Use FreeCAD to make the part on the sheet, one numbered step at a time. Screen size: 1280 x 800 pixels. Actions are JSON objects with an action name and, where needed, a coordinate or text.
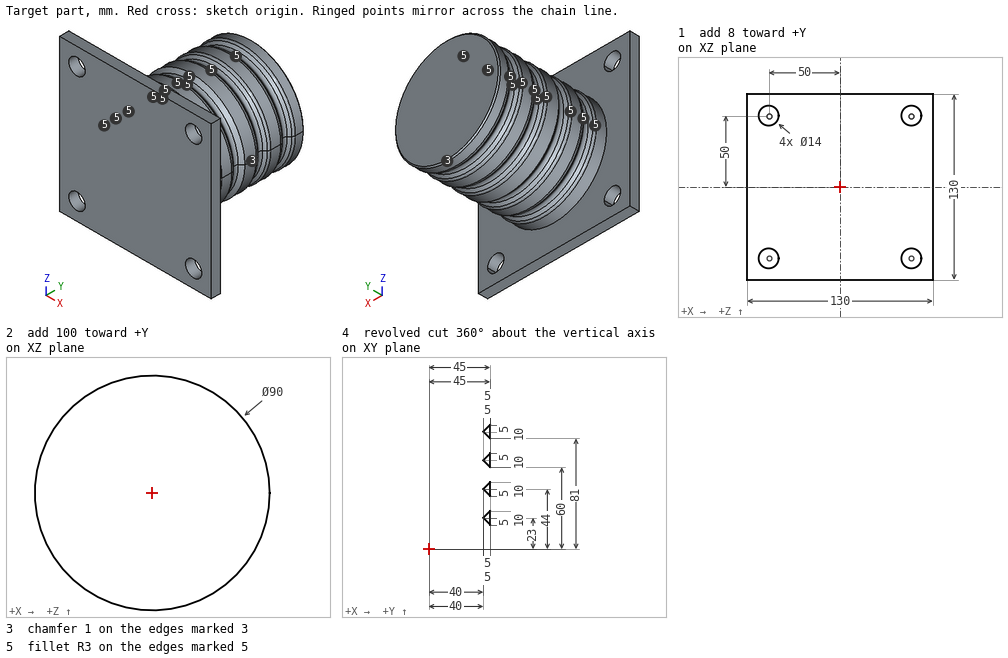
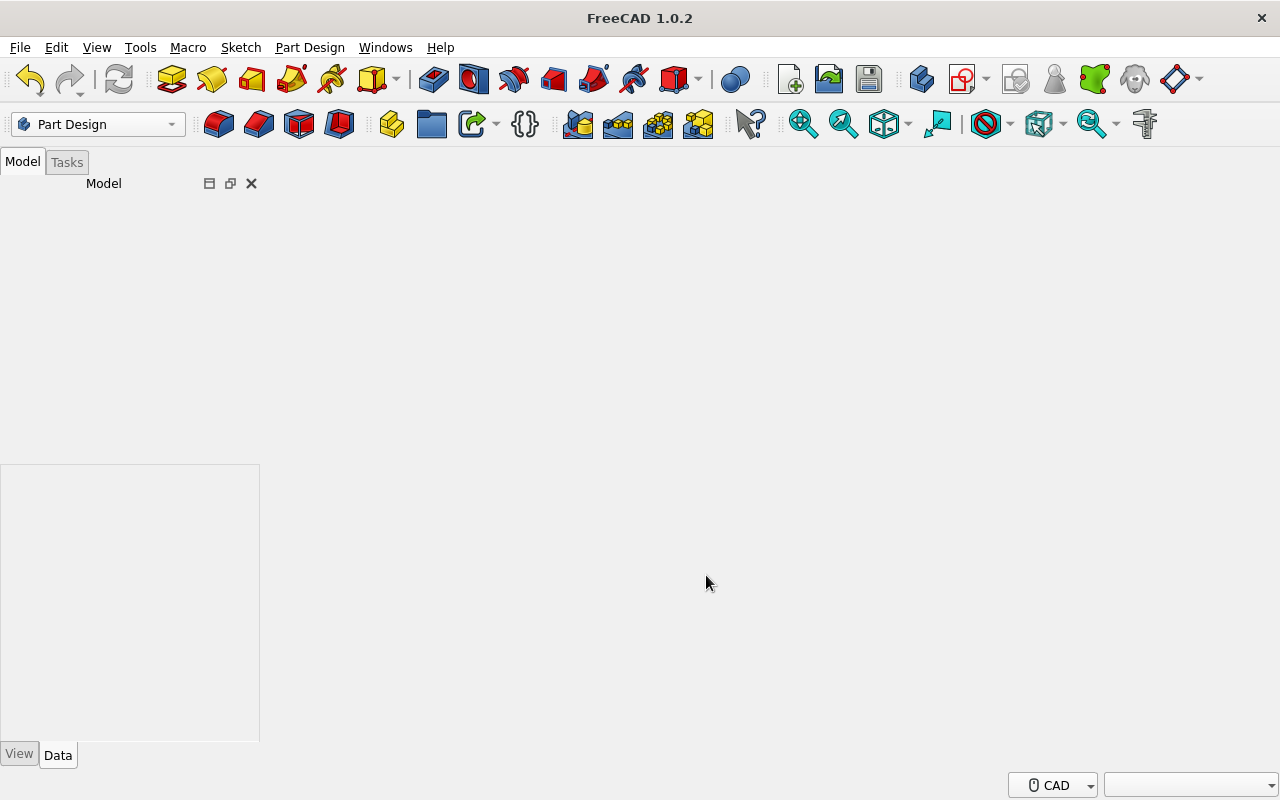
{"action": "left_click", "coordinate": [790, 80]}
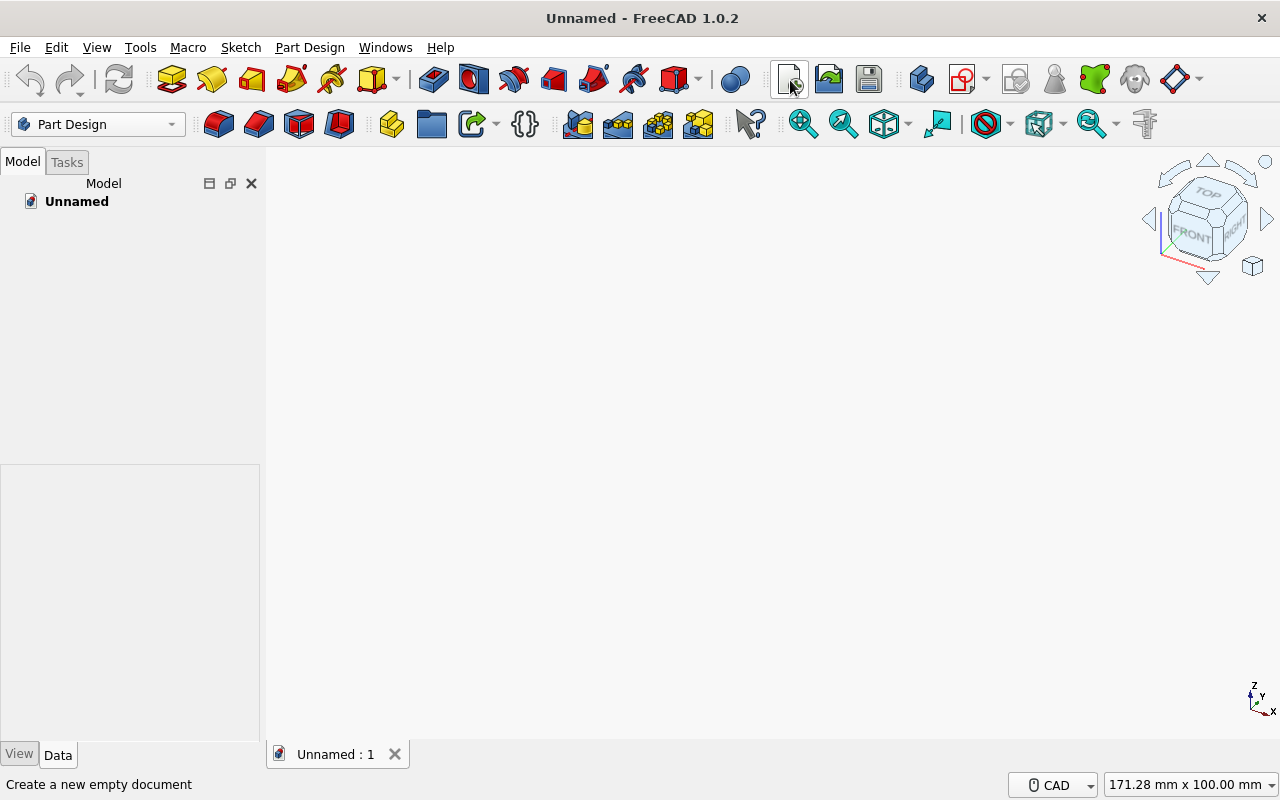
{"action": "left_click", "coordinate": [962, 80]}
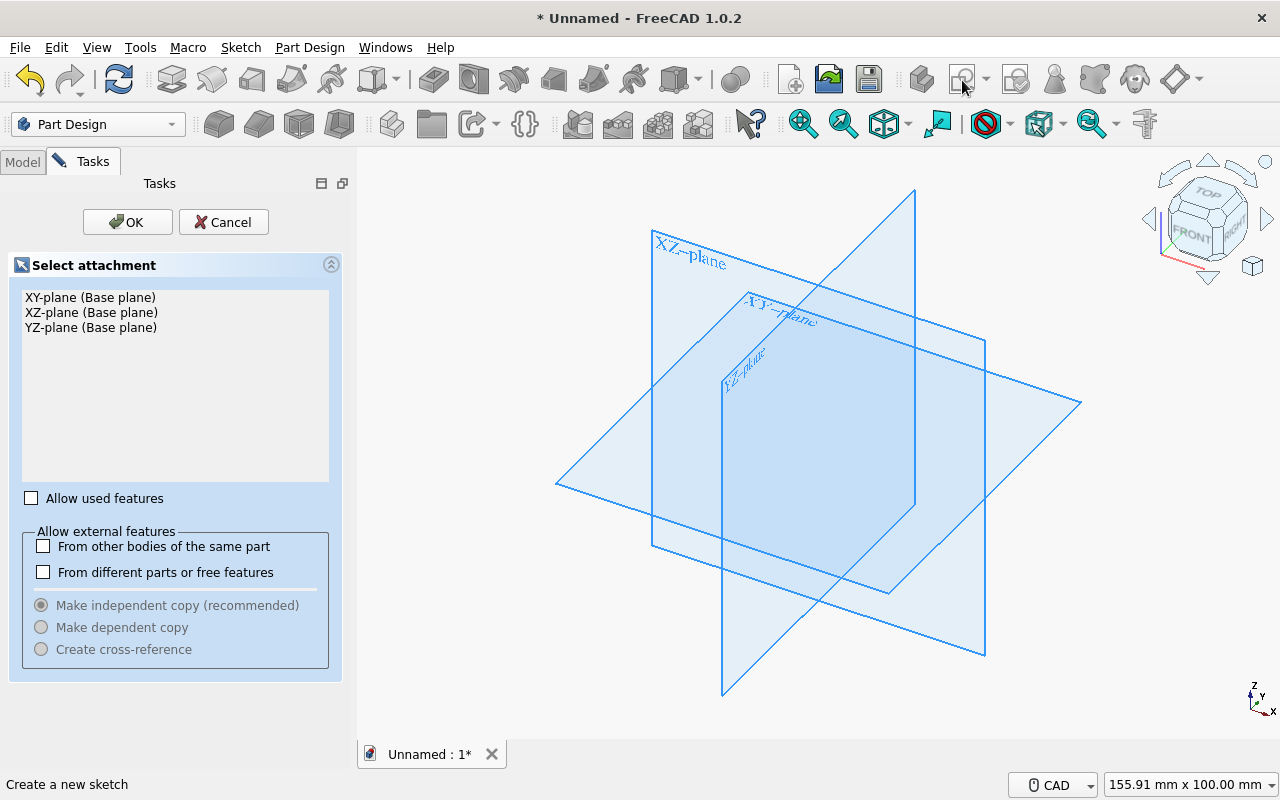
{"action": "left_click", "coordinate": [82, 312]}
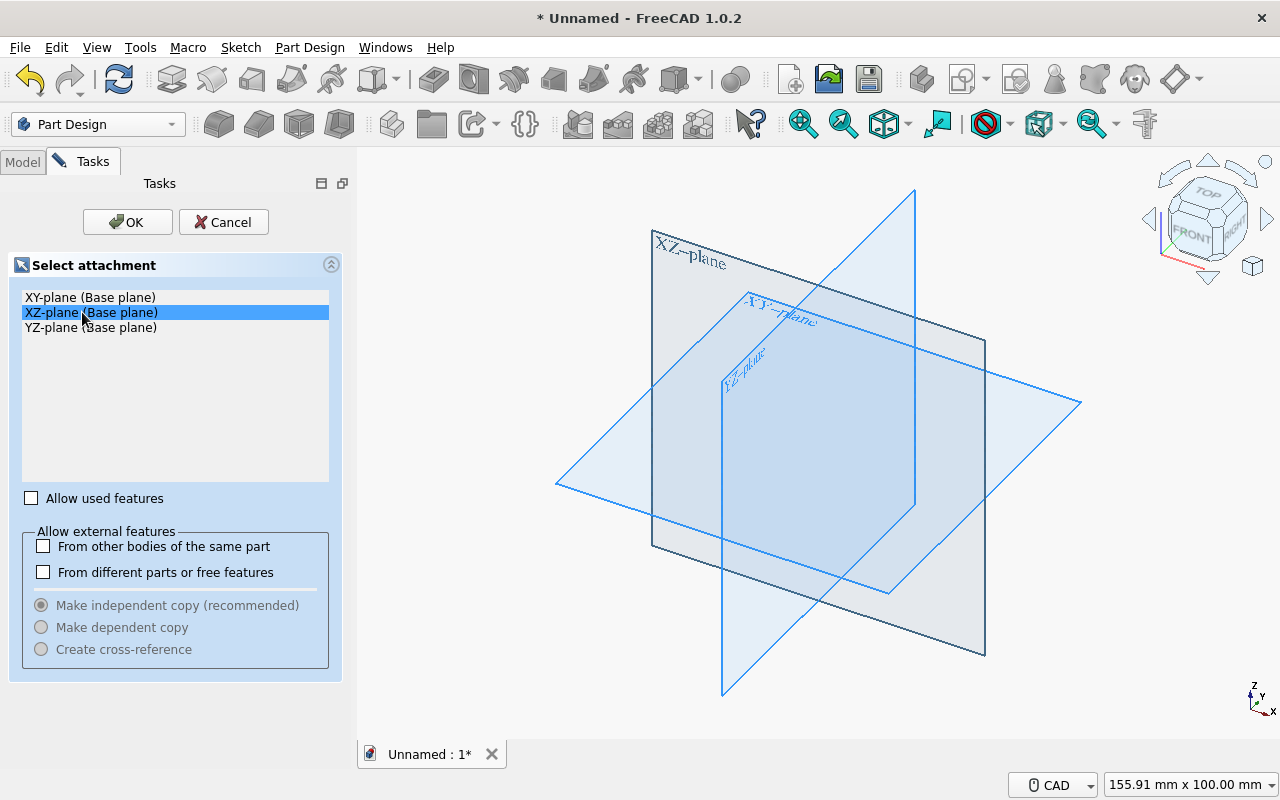
{"action": "left_click", "coordinate": [128, 222]}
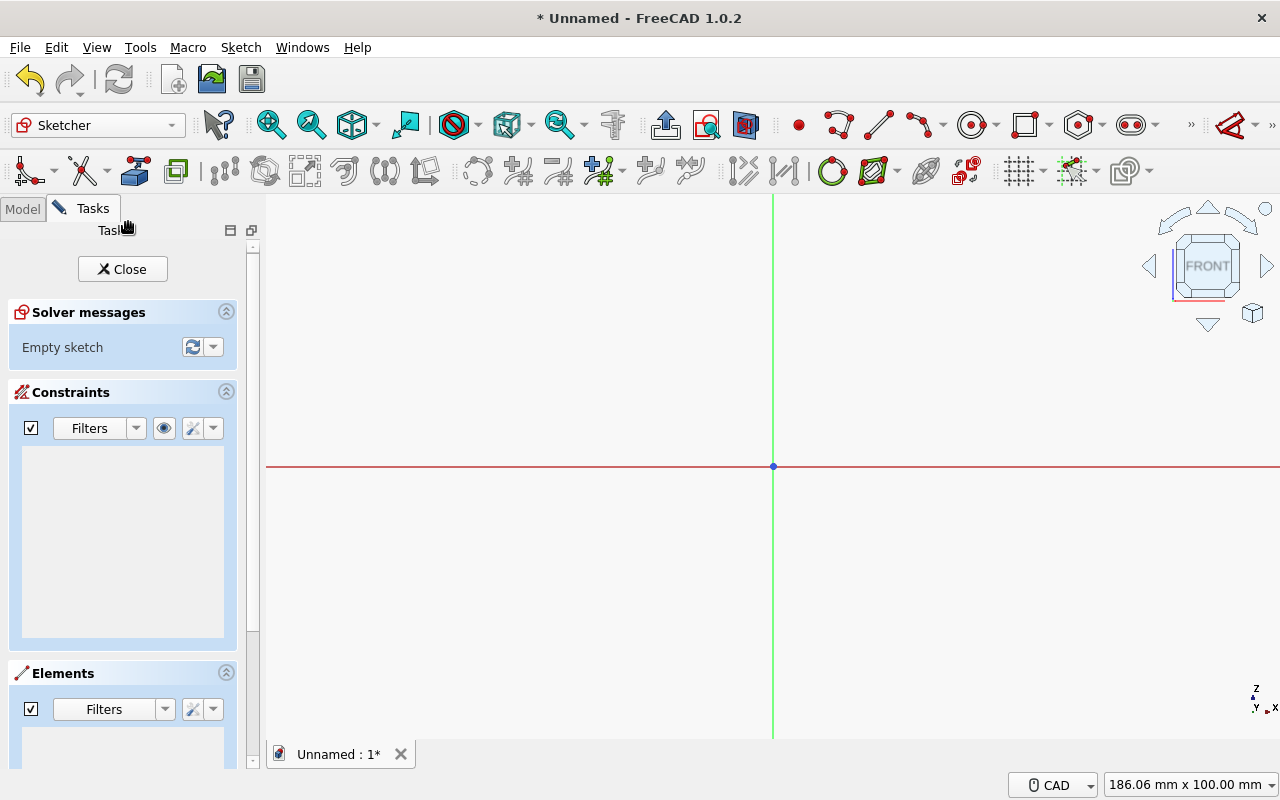
{"action": "scroll", "coordinate": [649, 466], "scroll_direction": "down", "scroll_amount": 4}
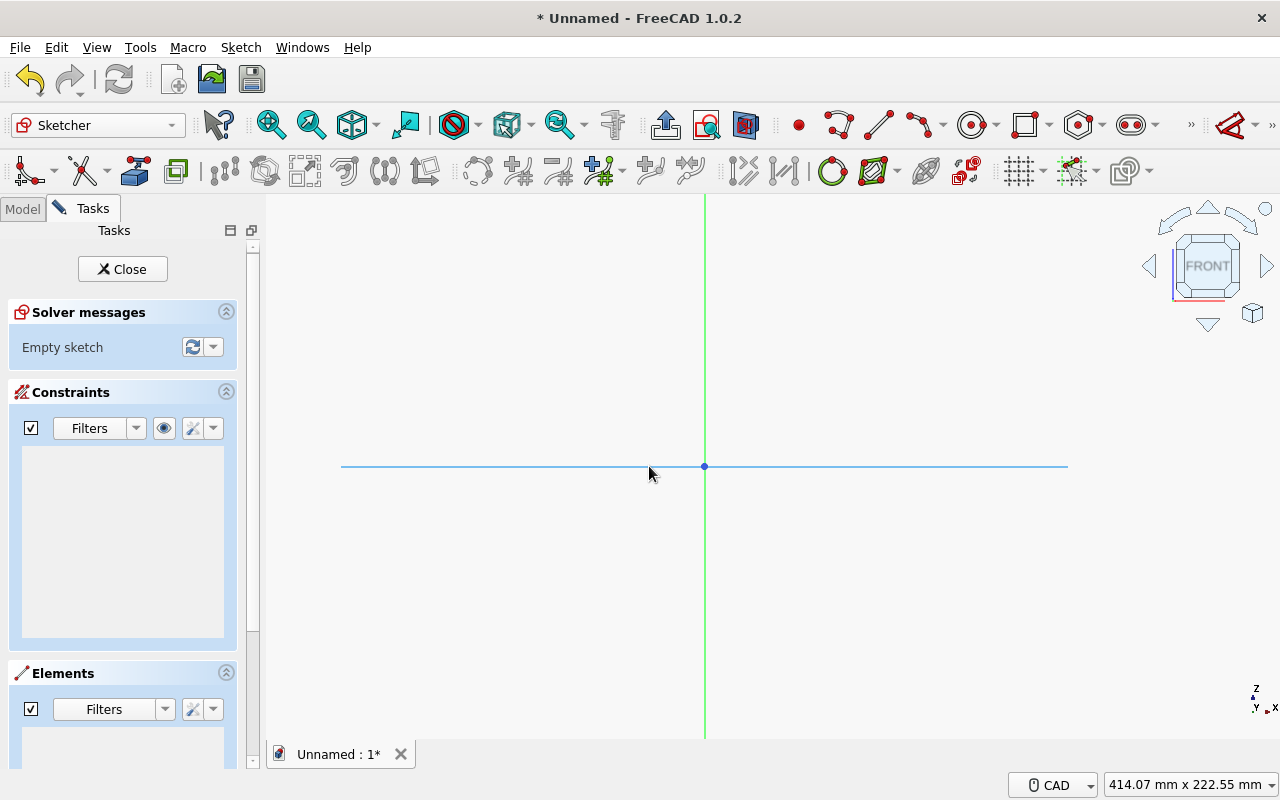
{"action": "left_click", "coordinate": [1052, 126]}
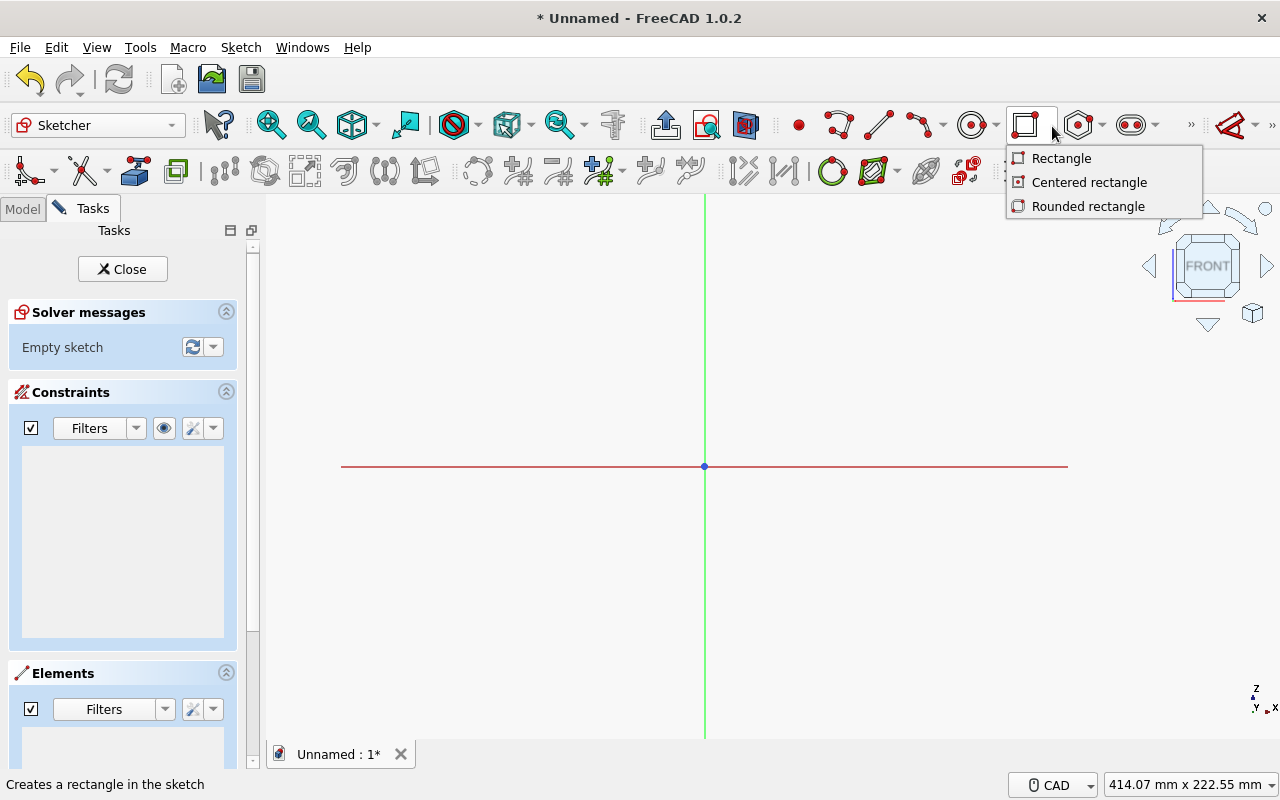
{"action": "left_click", "coordinate": [1104, 182]}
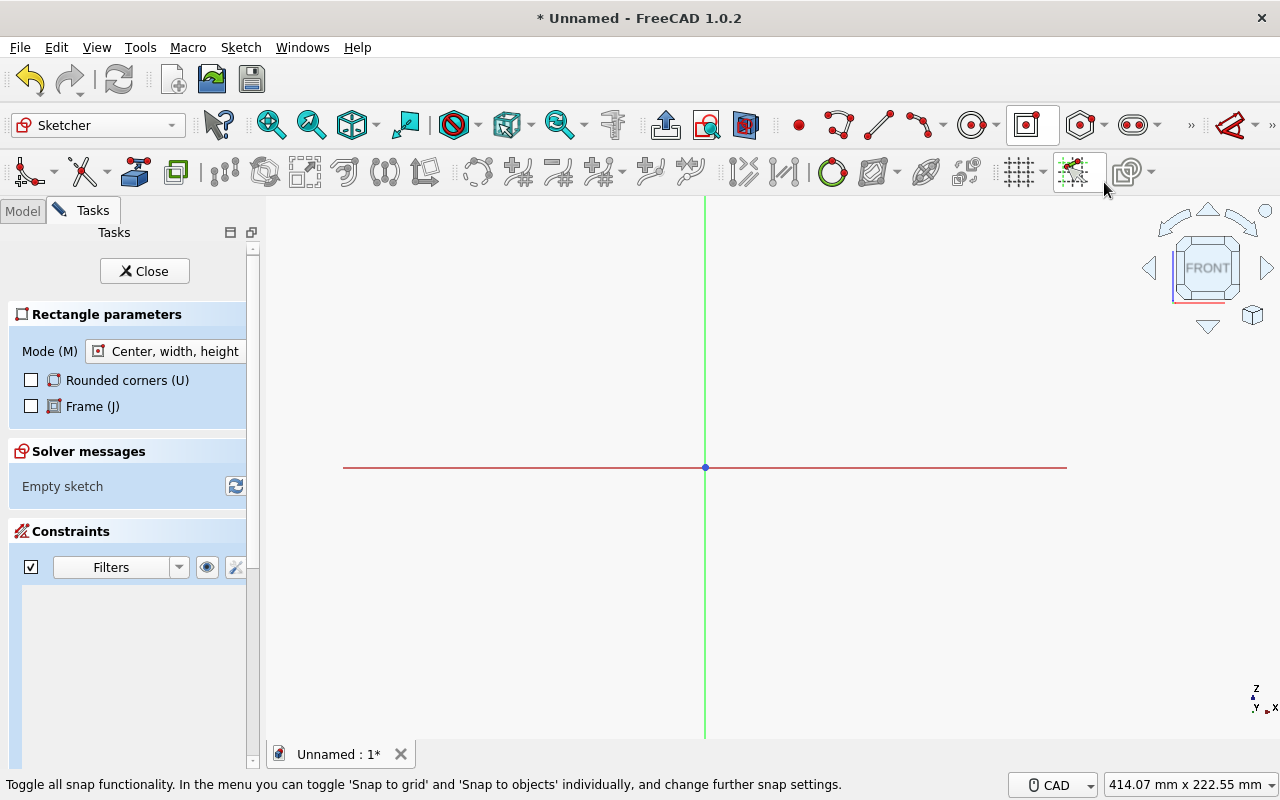
{"action": "left_click", "coordinate": [705, 468]}
{"action": "mouse_move", "coordinate": [864, 309]}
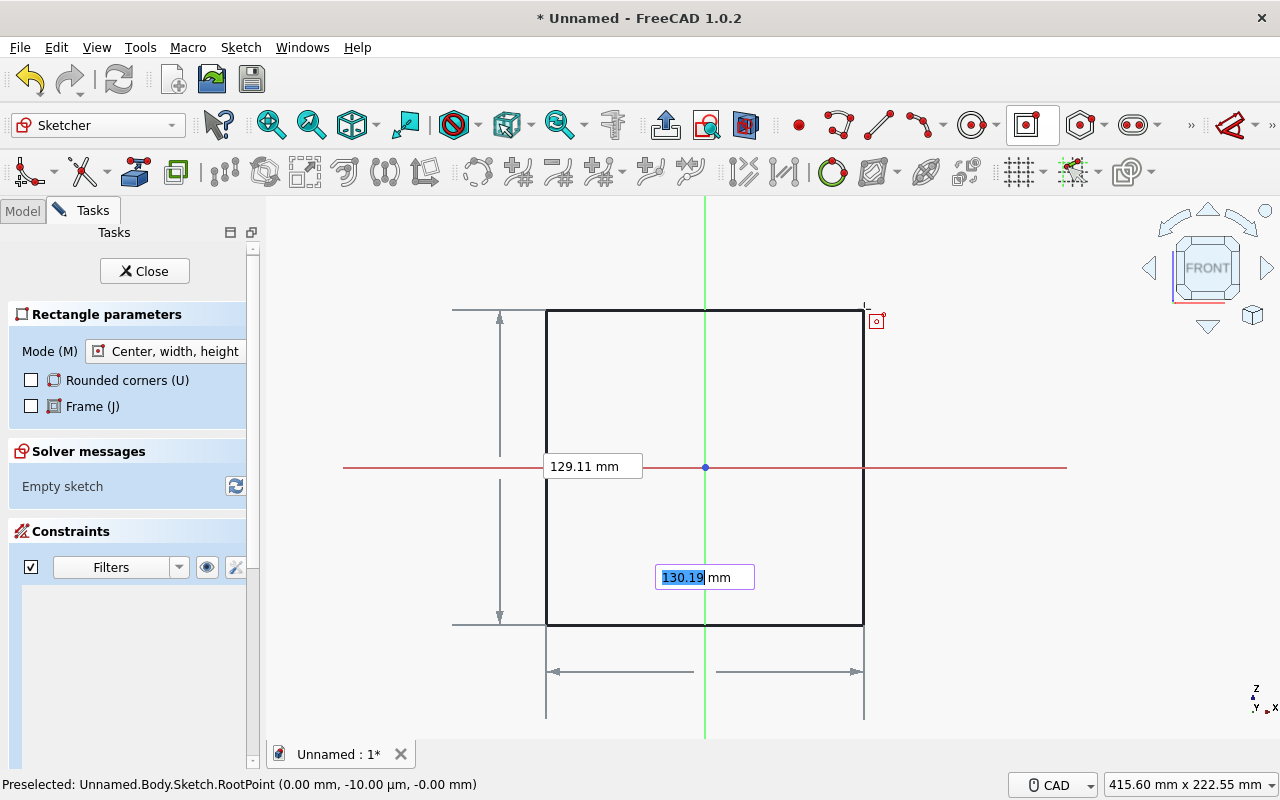
{"action": "type", "text": "130"}
{"action": "key", "text": "Tab"}
{"action": "type", "text": "130"}
{"action": "key", "text": "Return"}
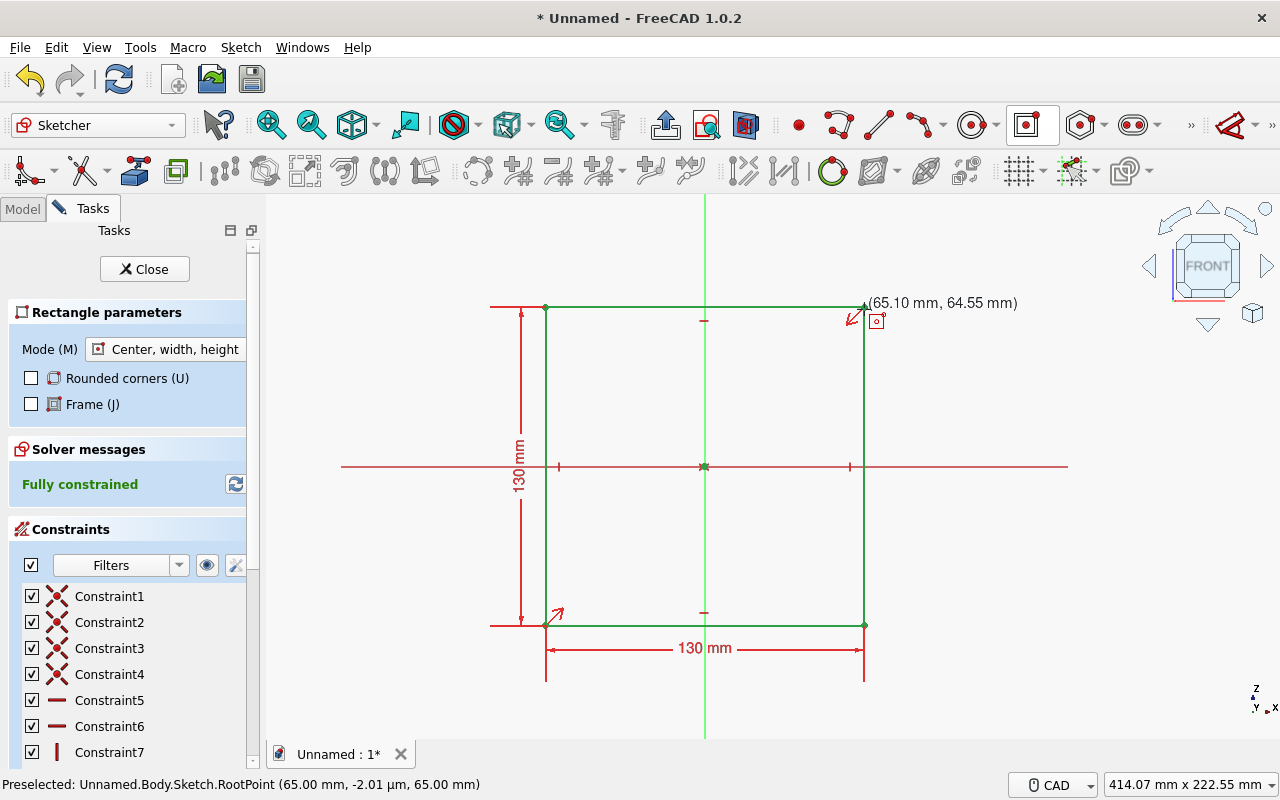
{"action": "left_click", "coordinate": [972, 126]}